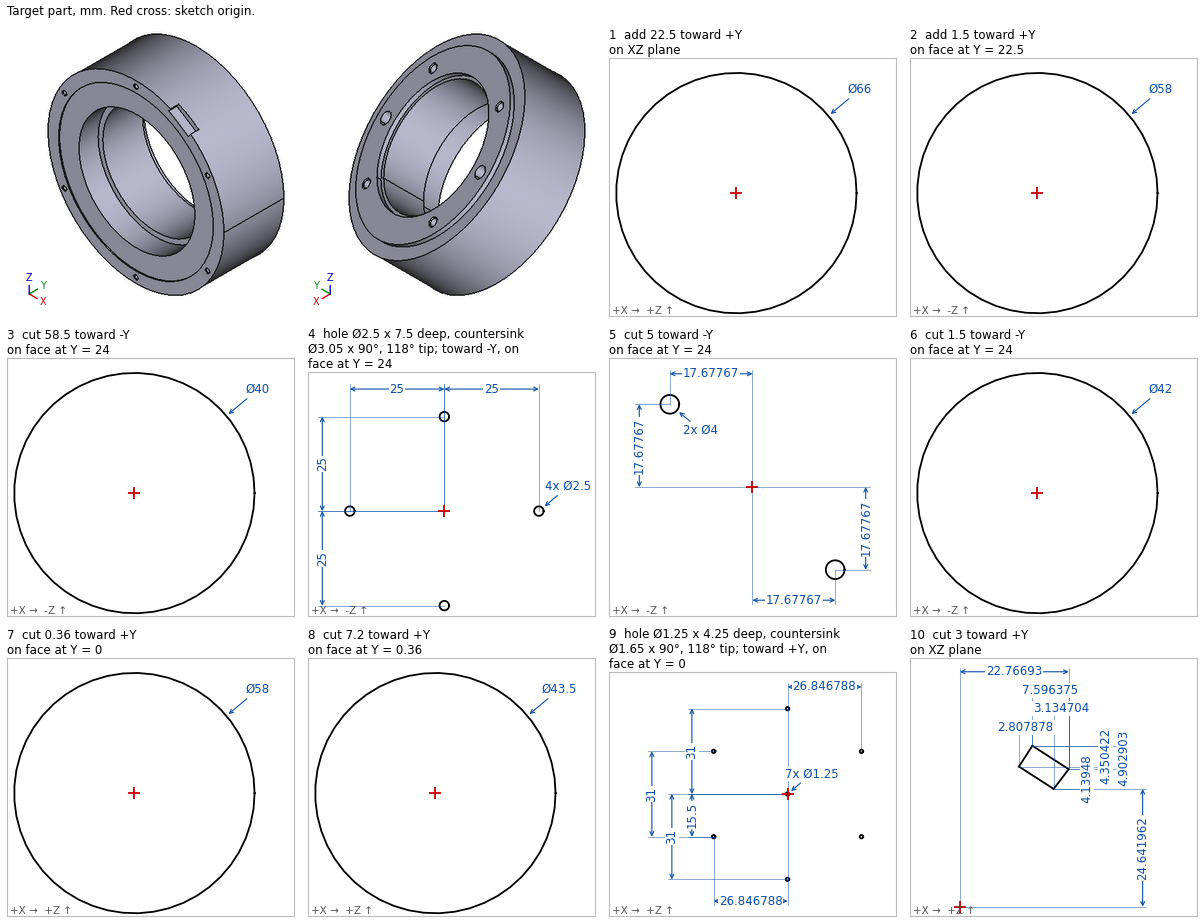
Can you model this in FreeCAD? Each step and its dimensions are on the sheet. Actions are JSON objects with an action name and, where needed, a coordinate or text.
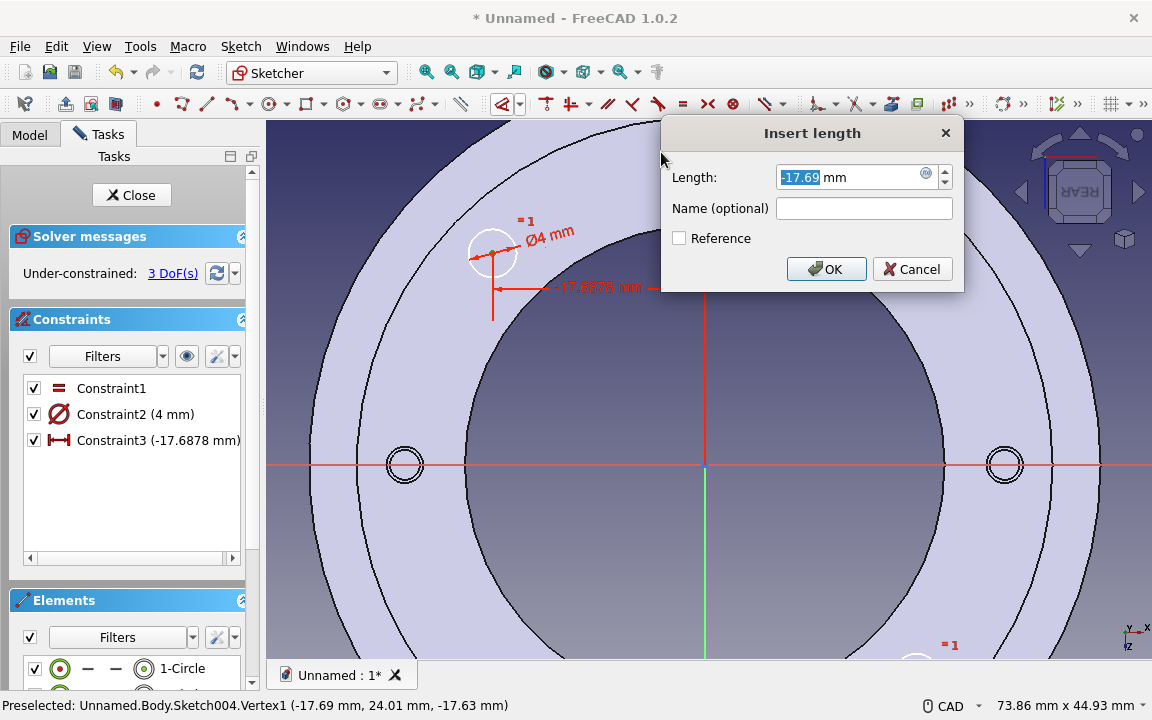
{"action": "type", "text": "-17.67767"}
{"action": "key", "text": "Return"}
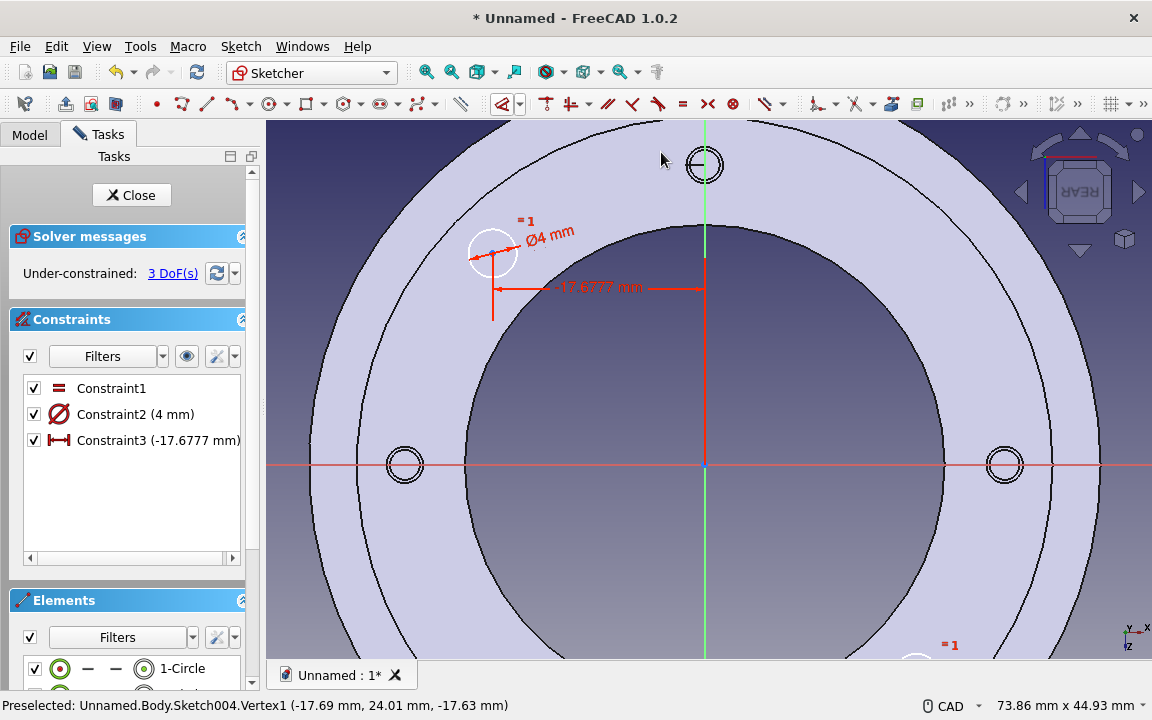
{"action": "left_click", "coordinate": [493, 253]}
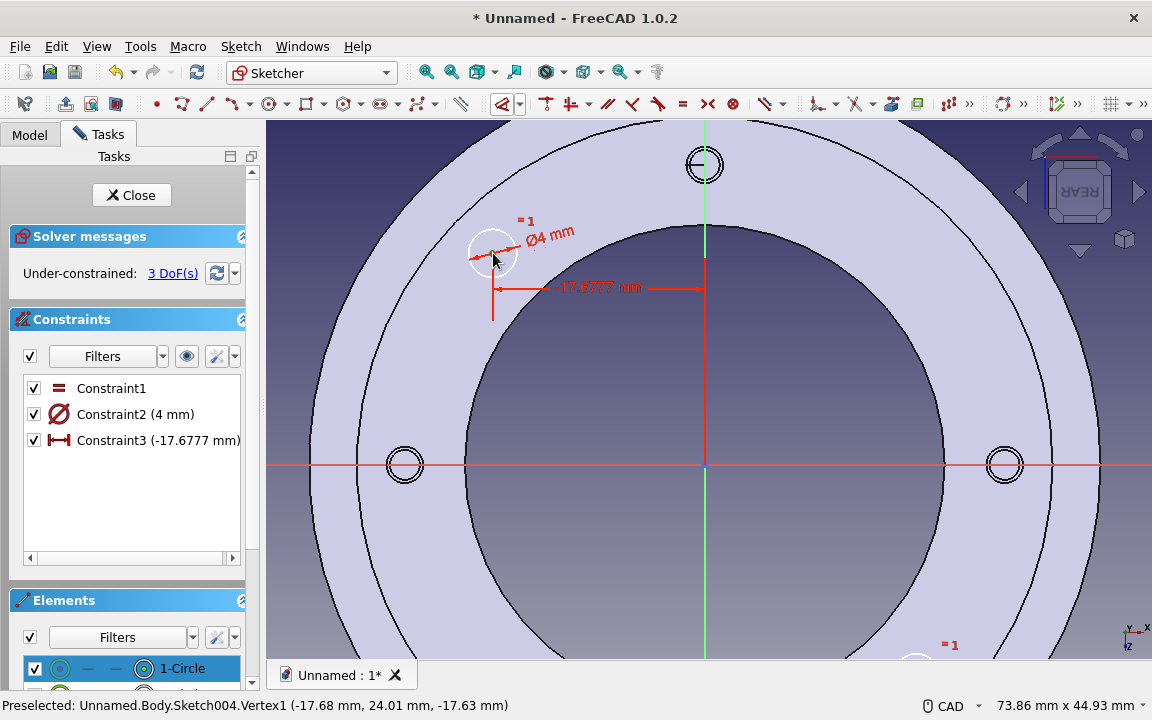
{"action": "key", "text": "i"}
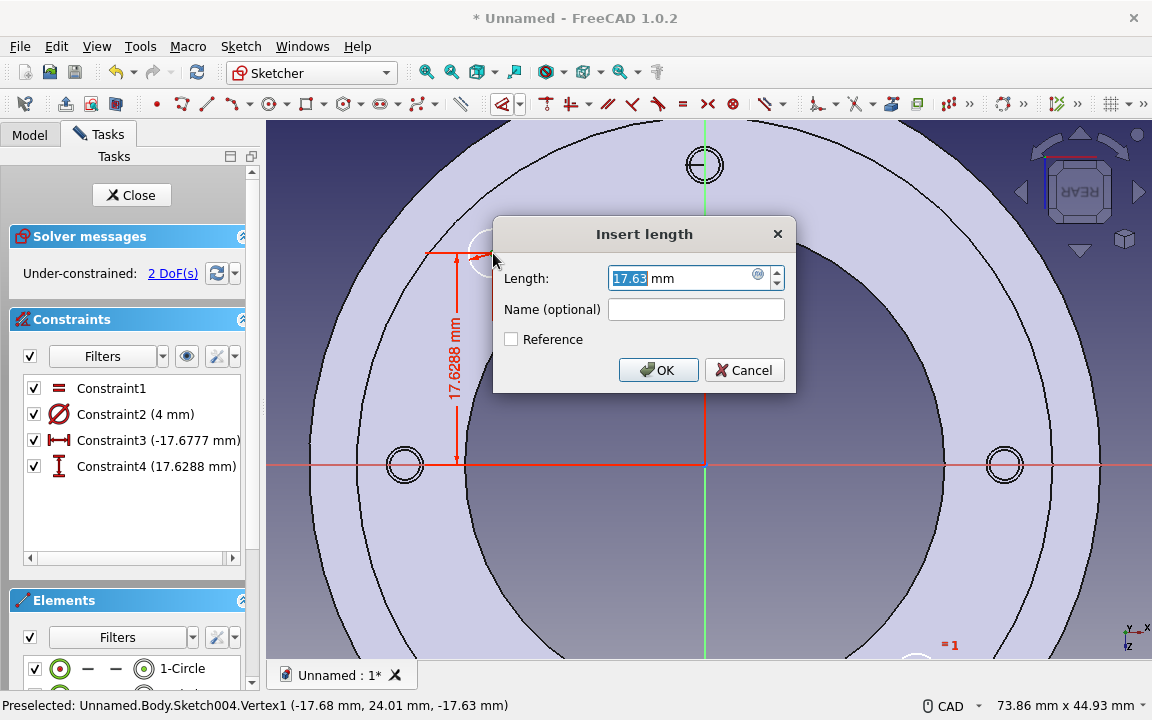
{"action": "type", "text": "17.67767"}
{"action": "key", "text": "Return"}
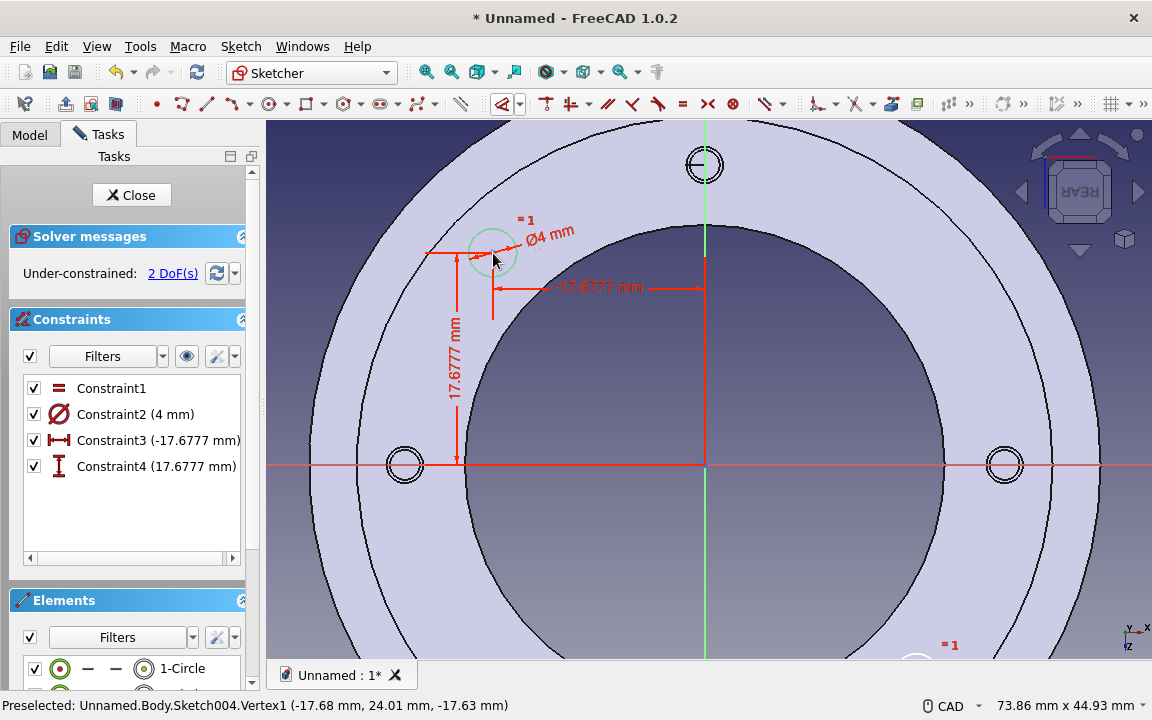
{"action": "scroll", "coordinate": [510, 236], "scroll_direction": "down", "scroll_amount": 2}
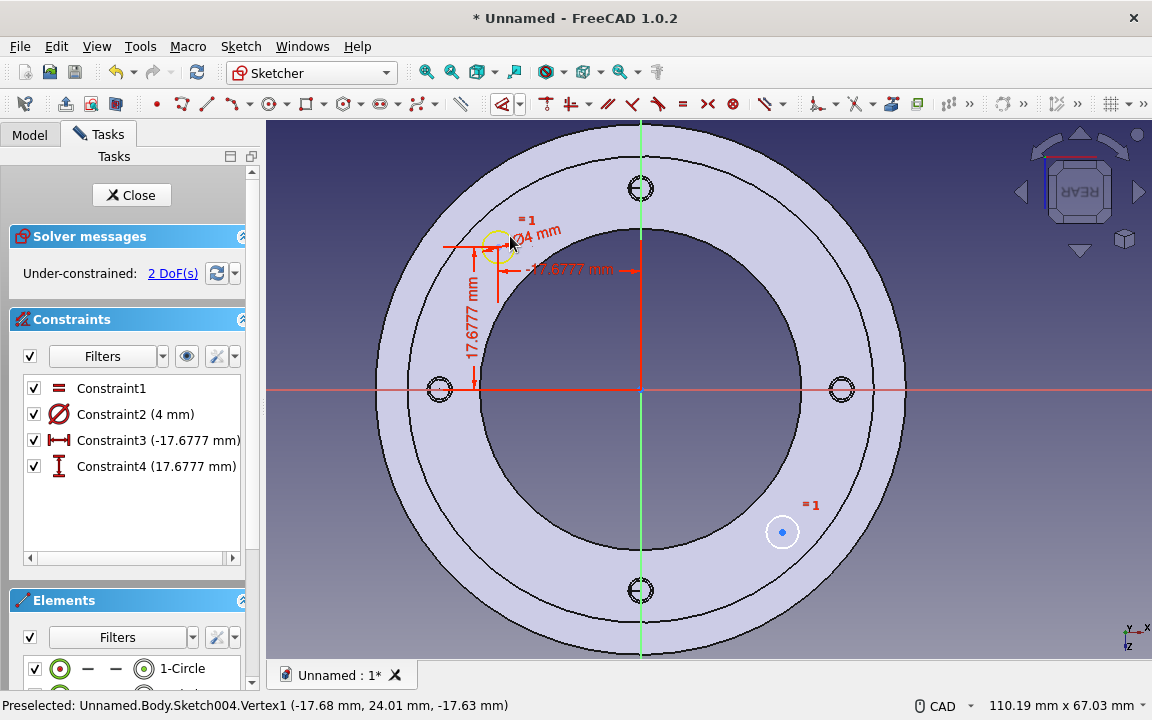
{"action": "left_click", "coordinate": [783, 532]}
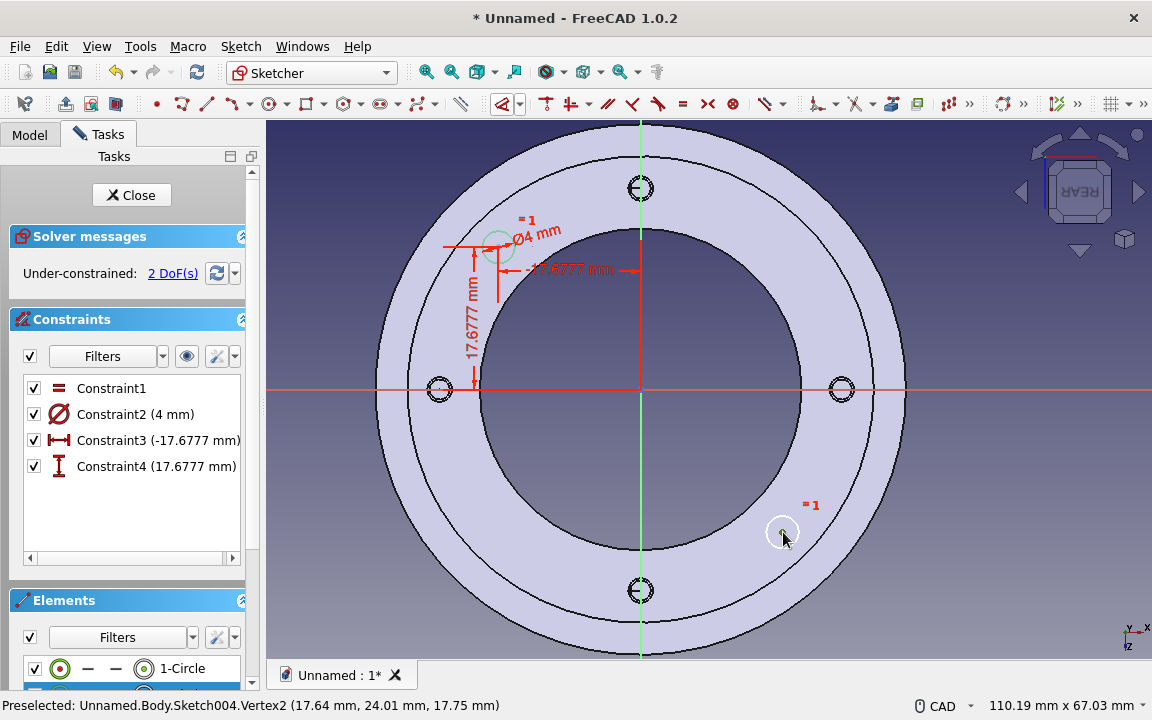
{"action": "key", "text": "l"}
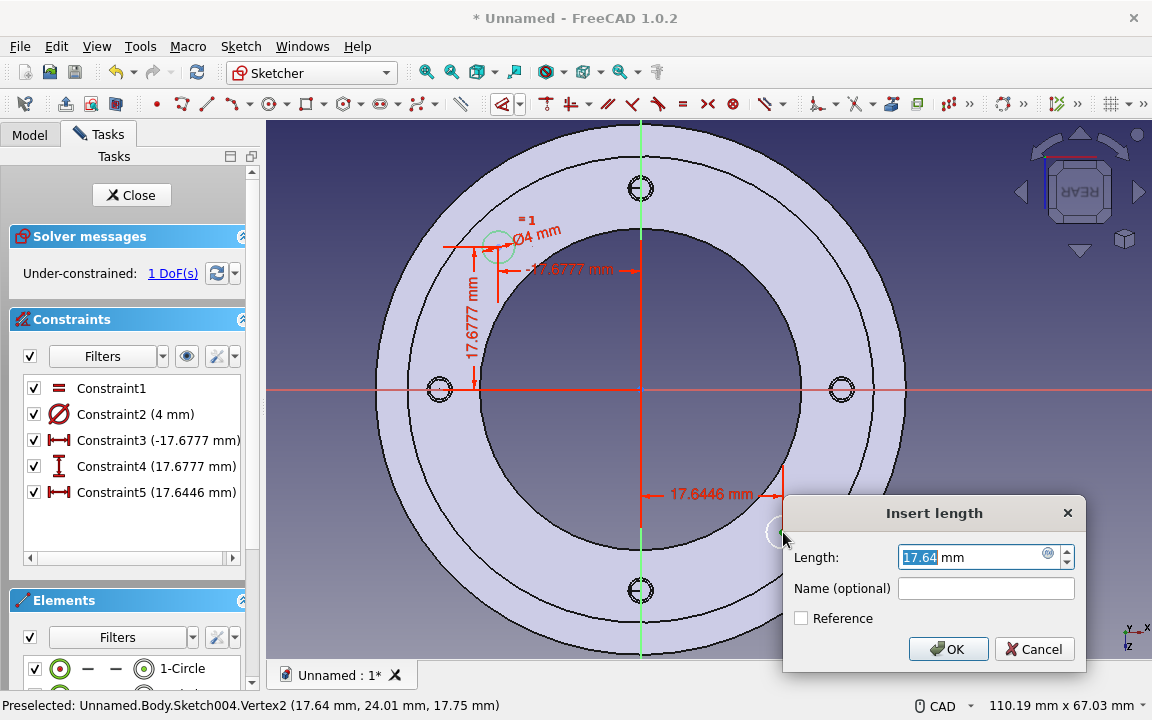
{"action": "type", "text": "17.67767"}
{"action": "key", "text": "Return"}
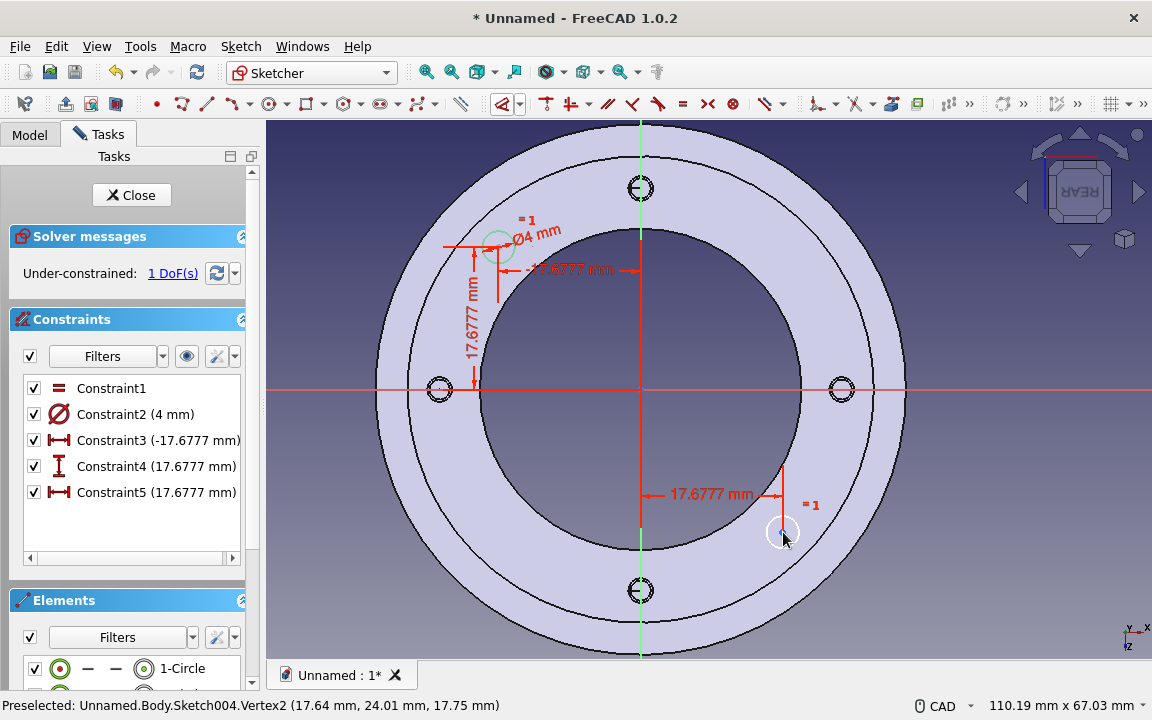
{"action": "left_click", "coordinate": [783, 532]}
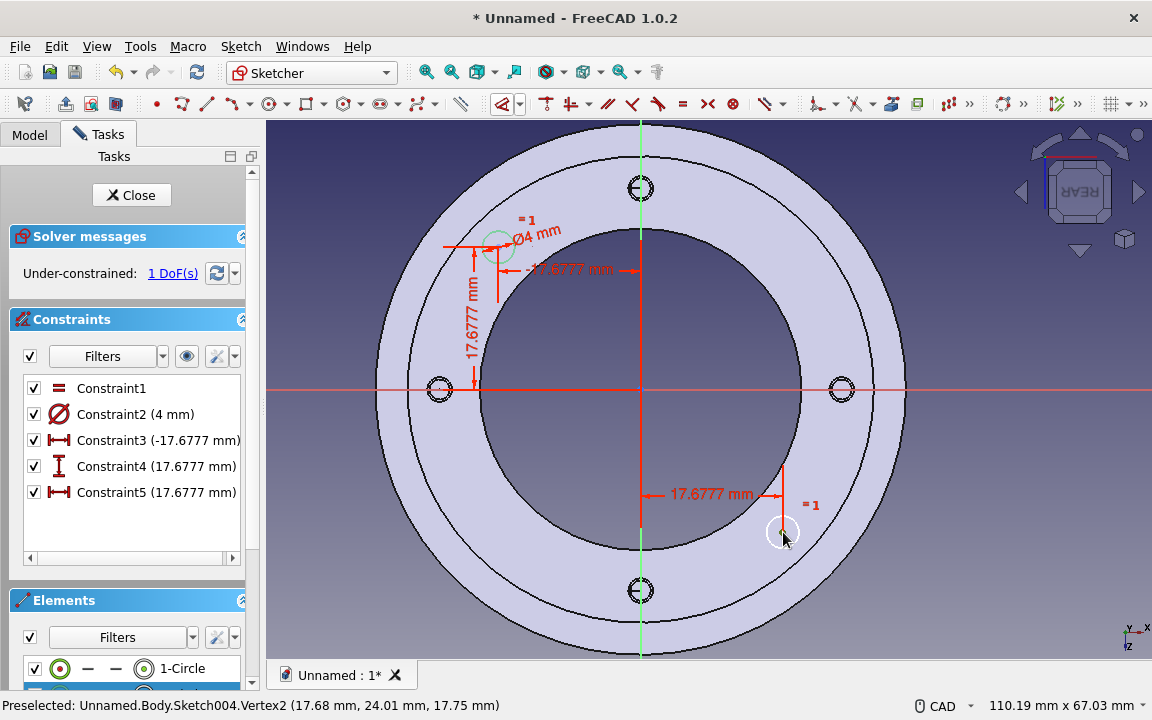
{"action": "left_click", "coordinate": [520, 104]}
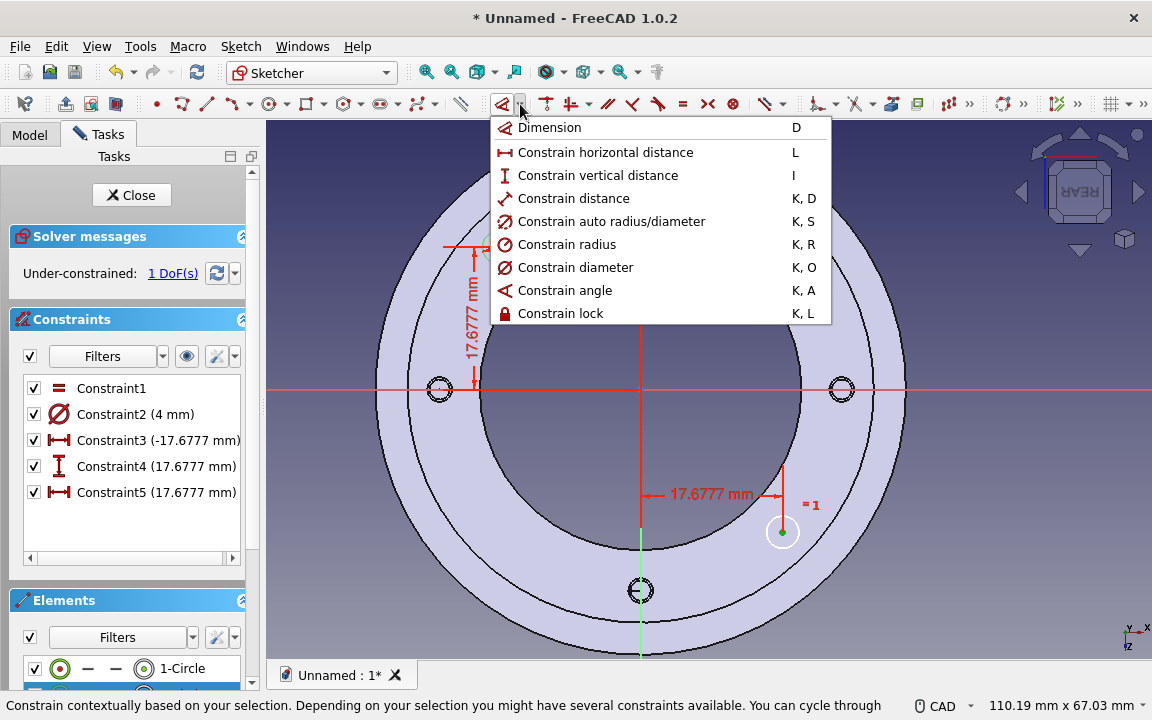
{"action": "left_click", "coordinate": [661, 176]}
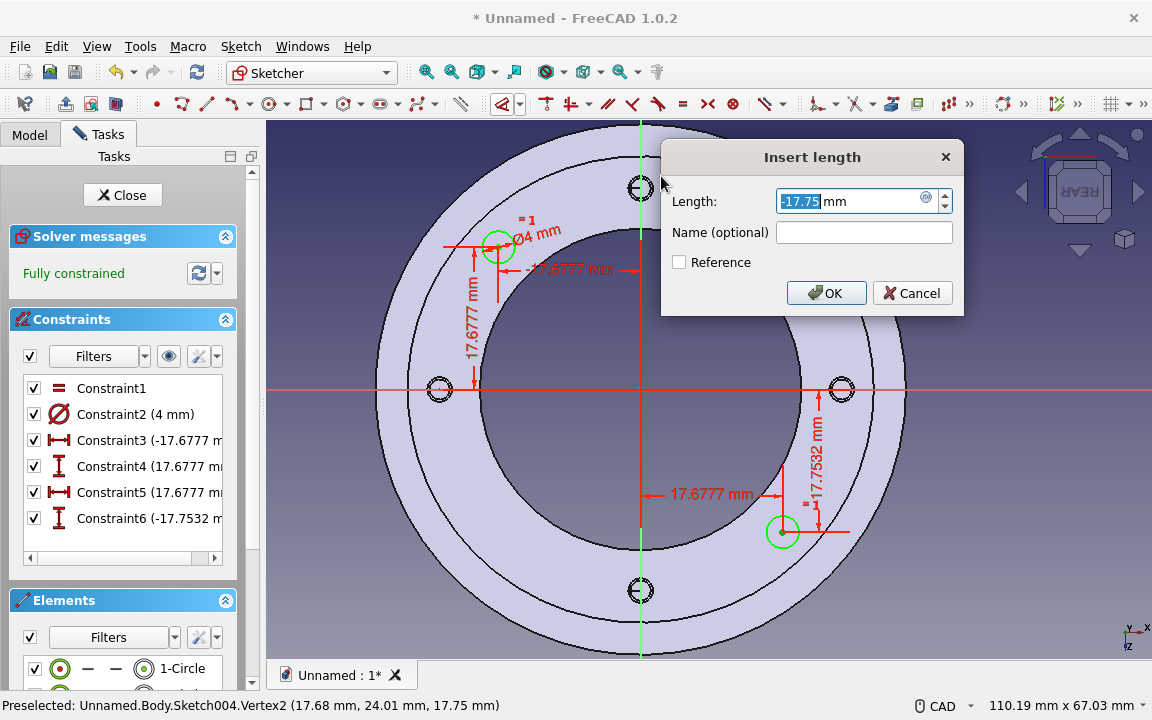
{"action": "type", "text": "-17.67767"}
{"action": "key", "text": "Return"}